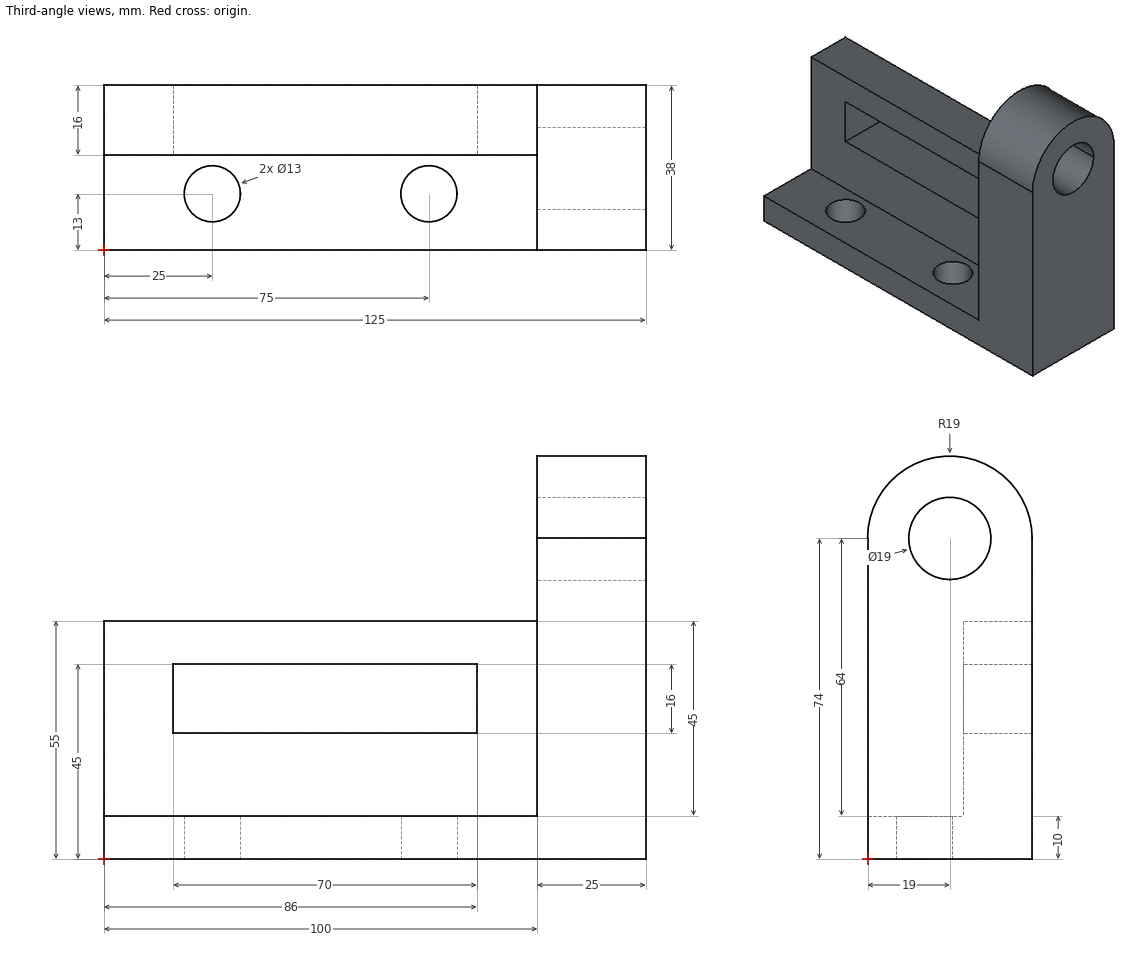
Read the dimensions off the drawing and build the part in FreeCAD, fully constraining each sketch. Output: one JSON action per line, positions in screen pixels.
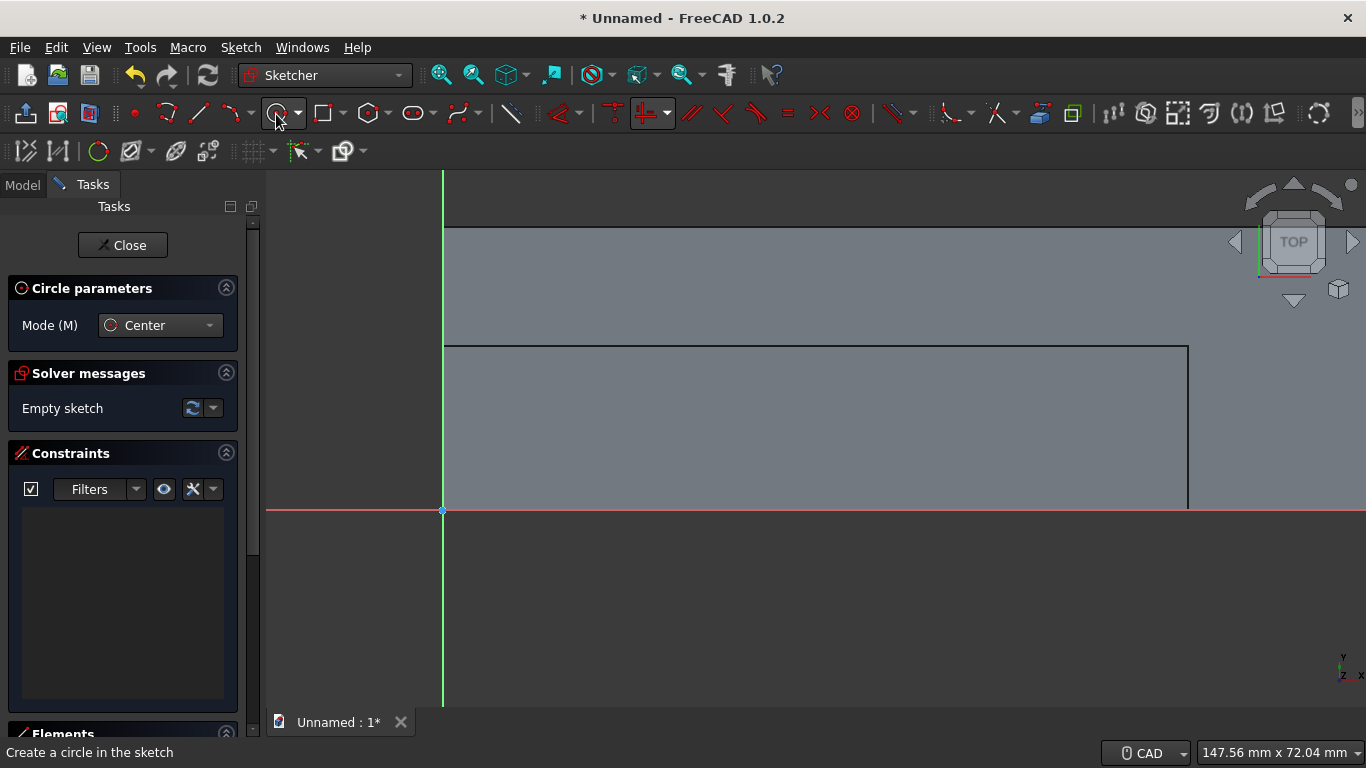
{"action": "left_click", "coordinate": [629, 413]}
{"action": "left_click", "coordinate": [663, 379]}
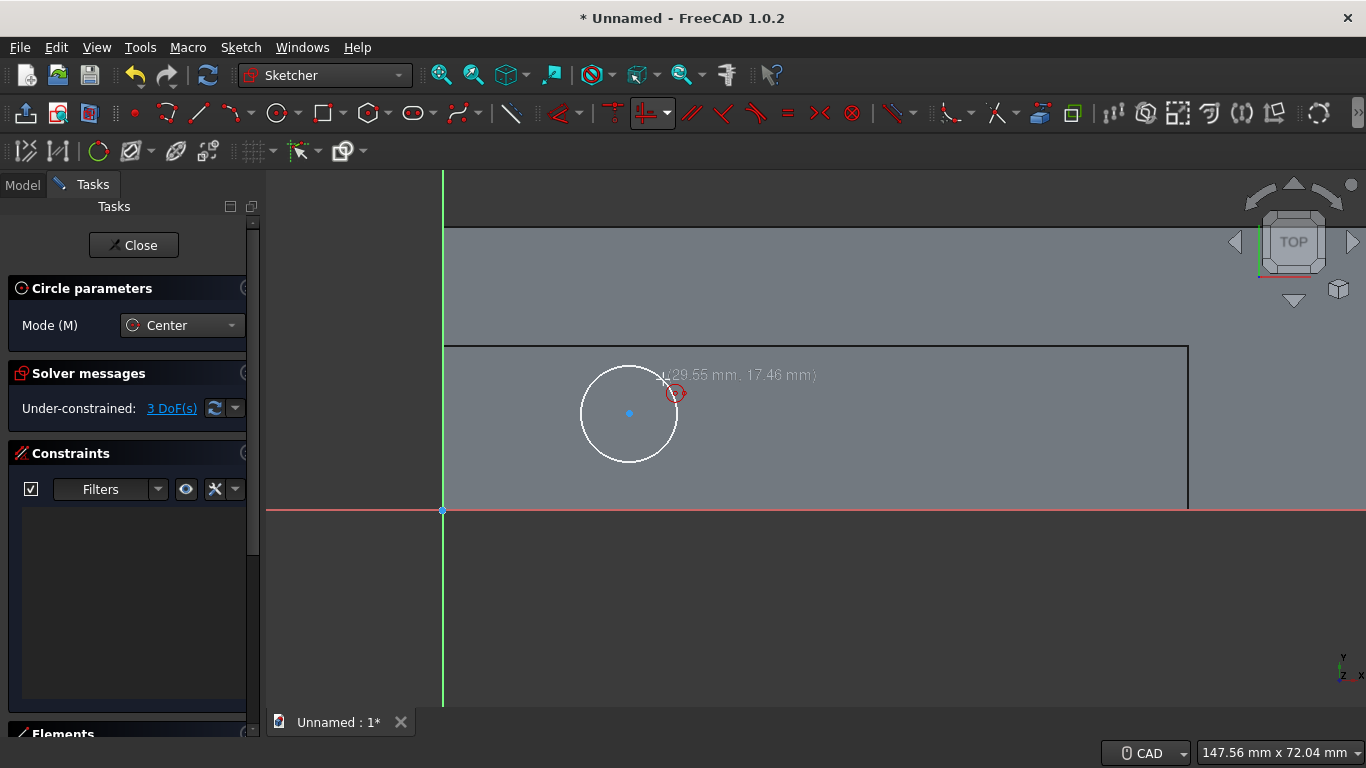
{"action": "left_click", "coordinate": [1002, 413]}
{"action": "left_click", "coordinate": [1036, 379]}
{"action": "key", "text": "Escape"}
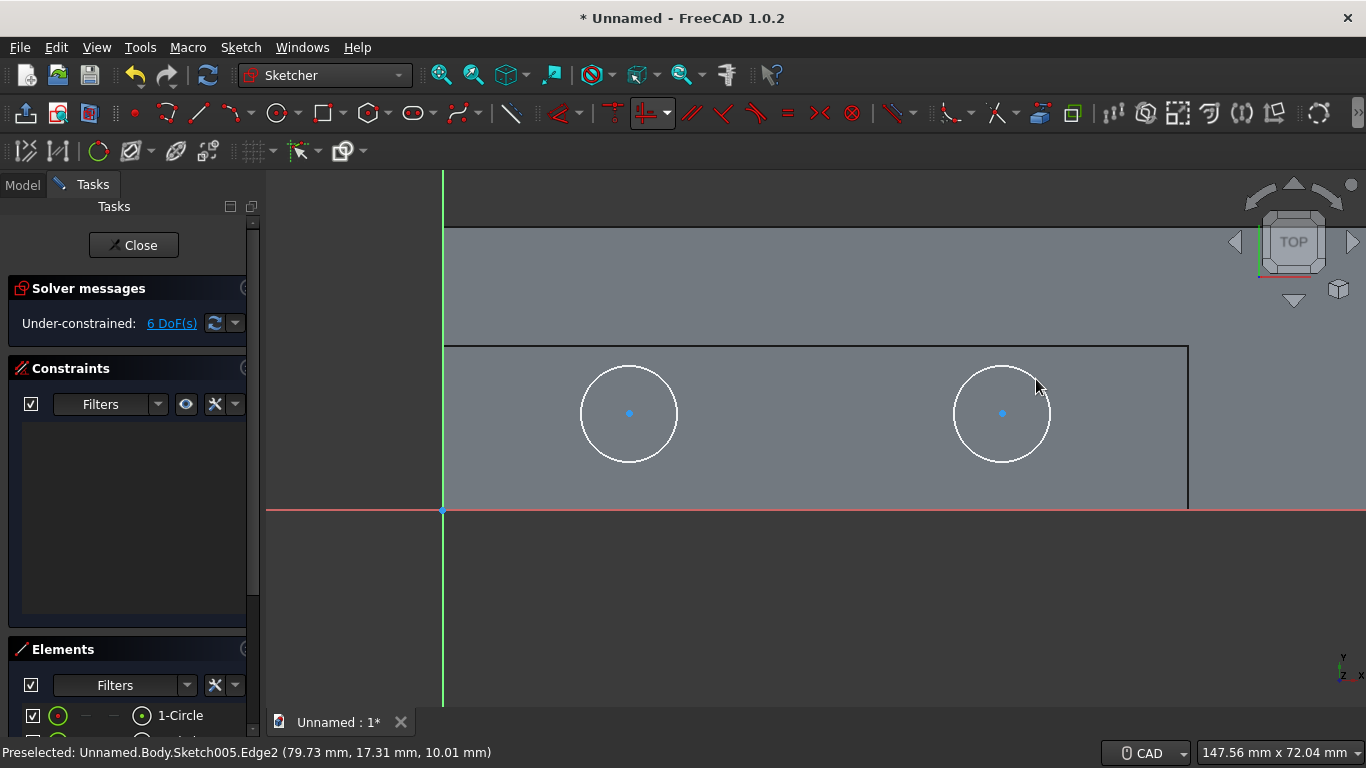
{"action": "left_click", "coordinate": [663, 380]}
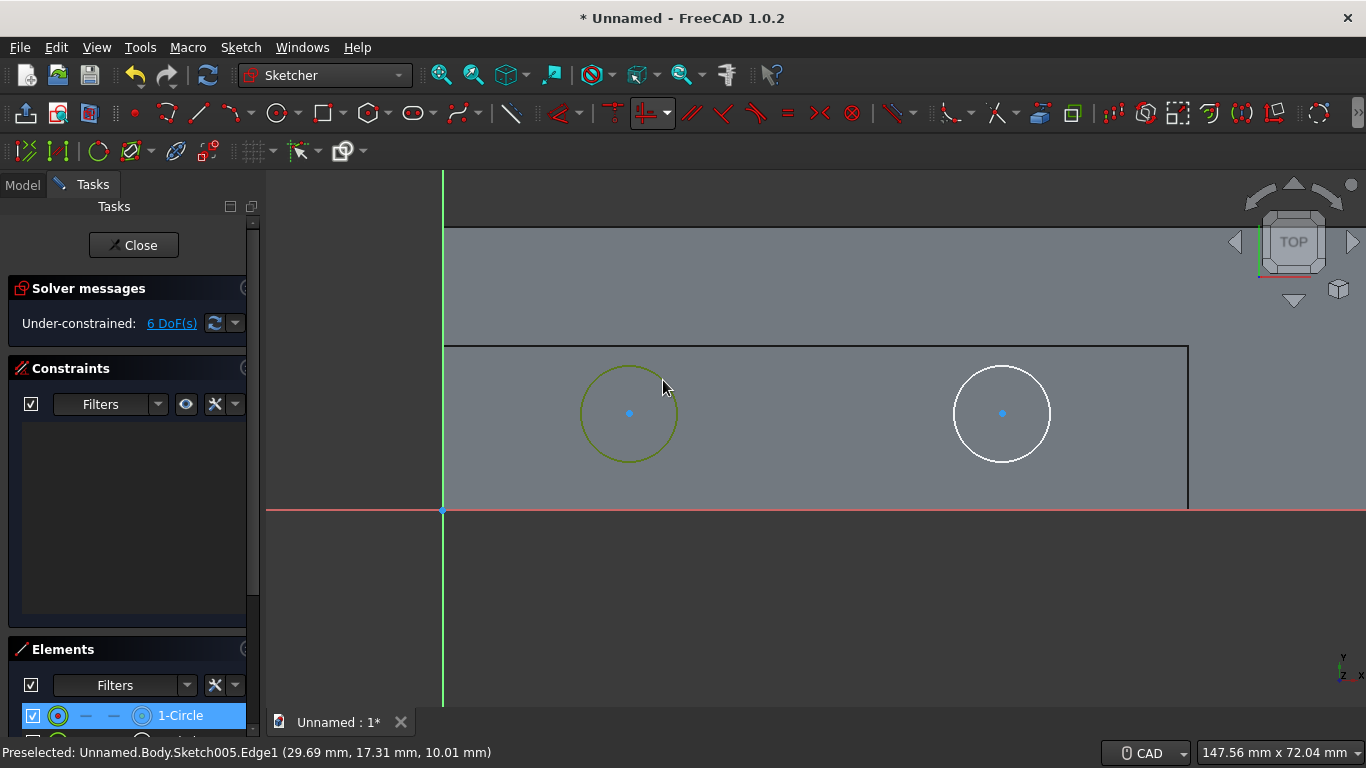
{"action": "left_click", "coordinate": [1036, 380]}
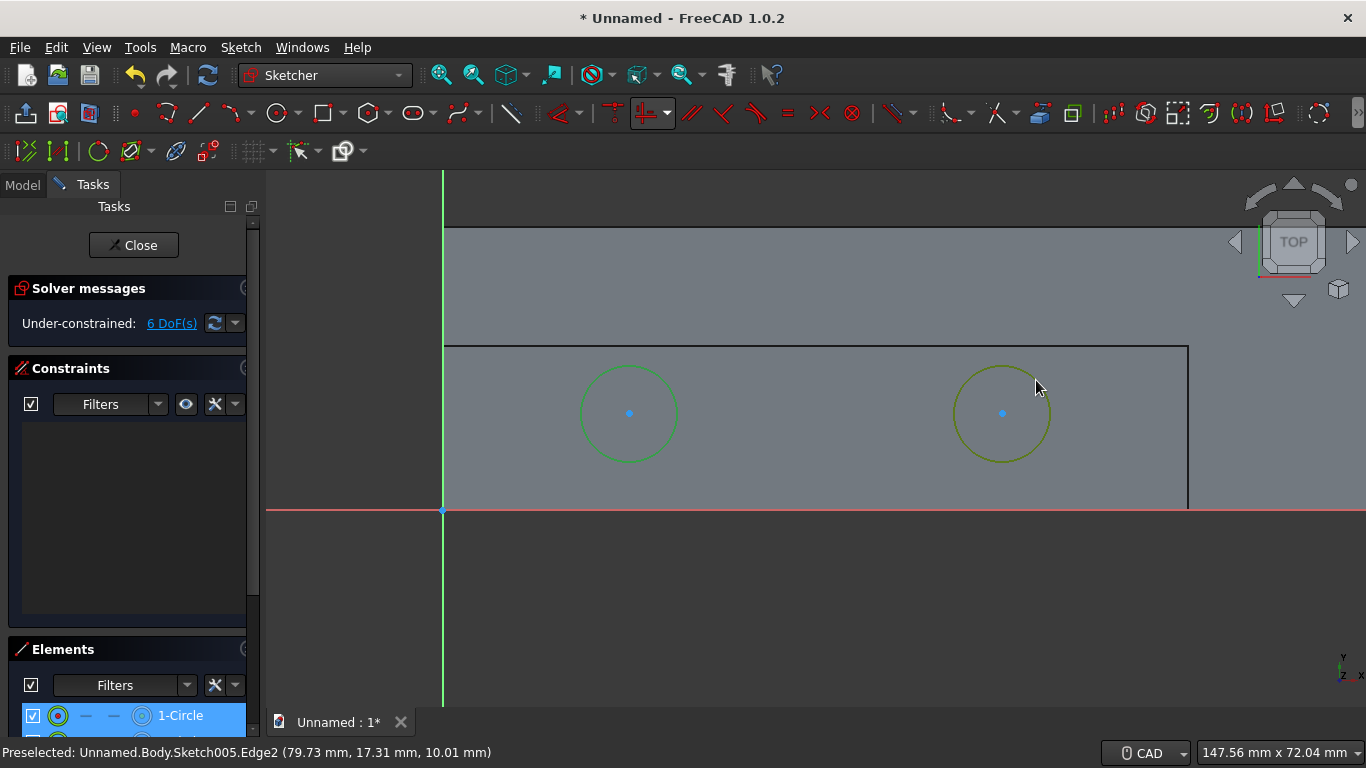
{"action": "left_click", "coordinate": [788, 114]}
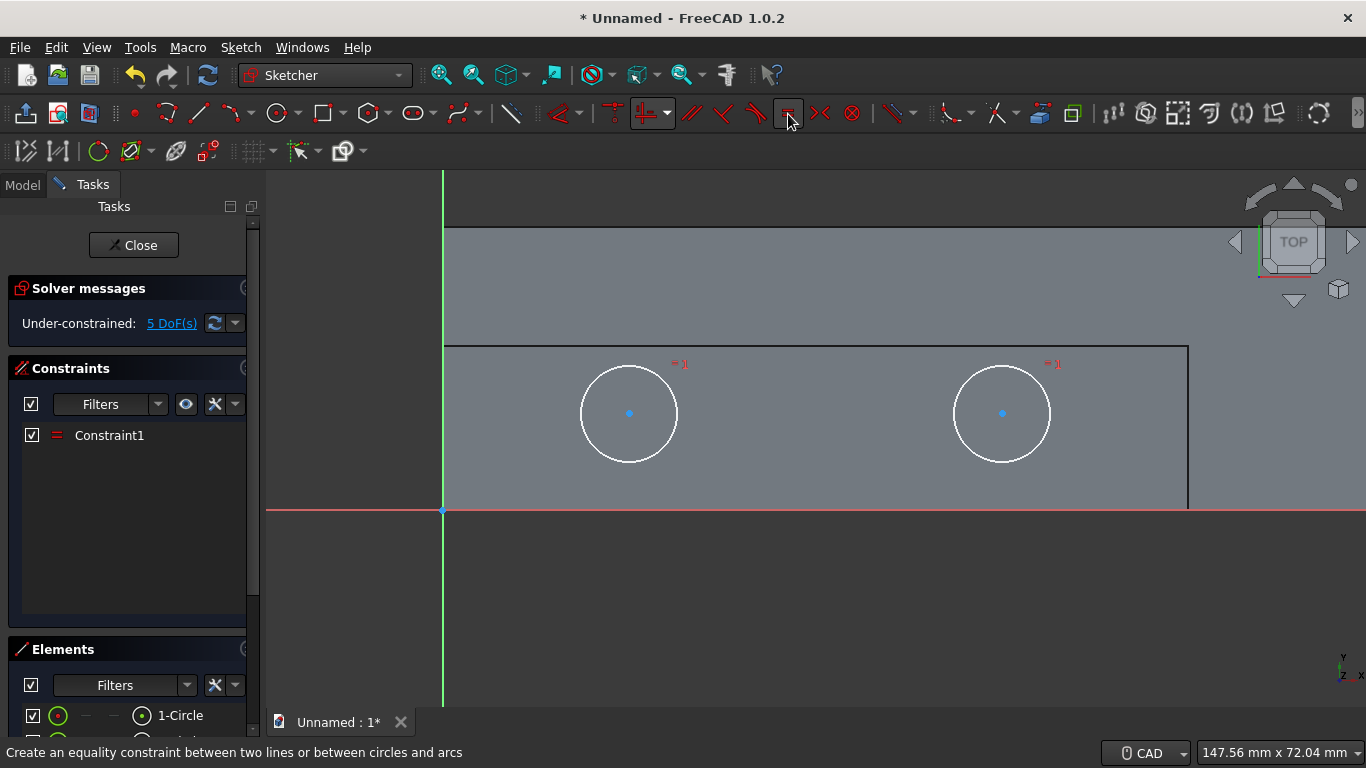
{"action": "left_click", "coordinate": [629, 414]}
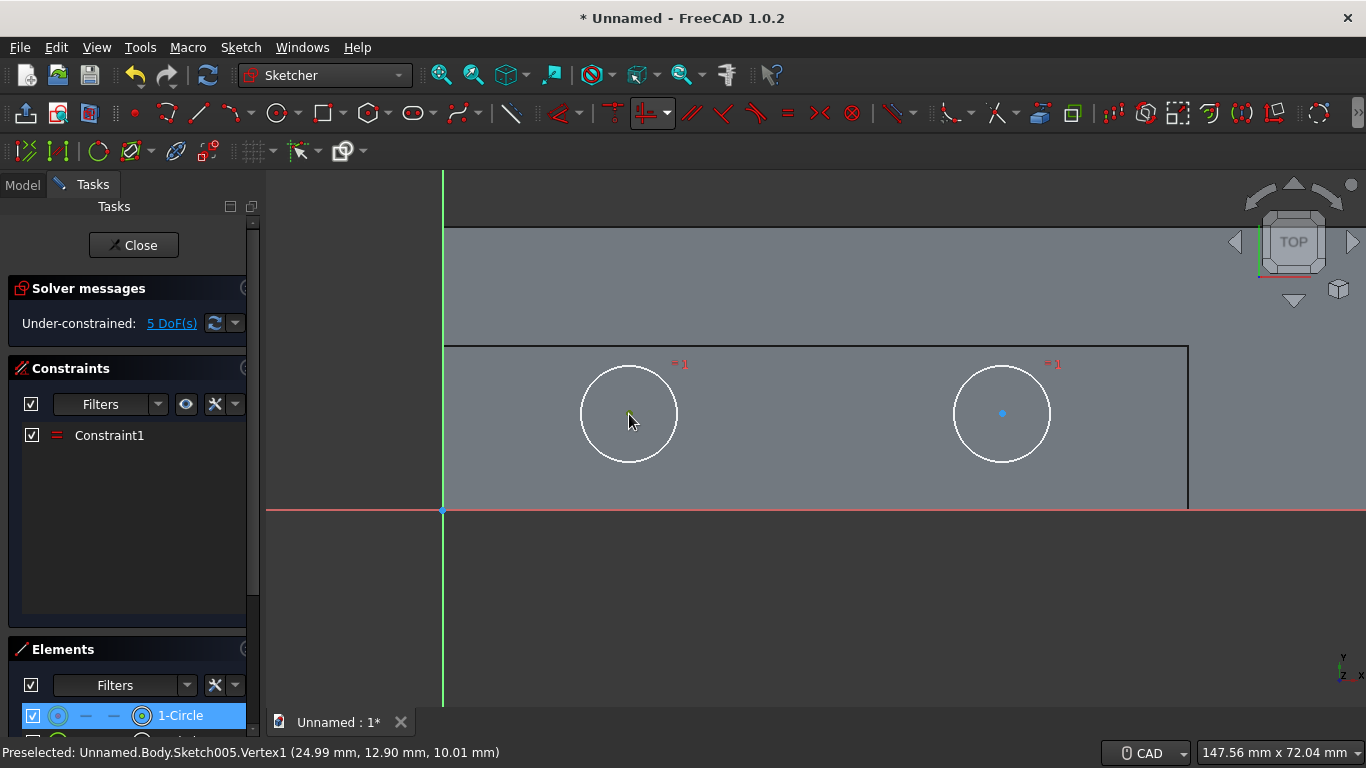
{"action": "left_click", "coordinate": [1002, 414]}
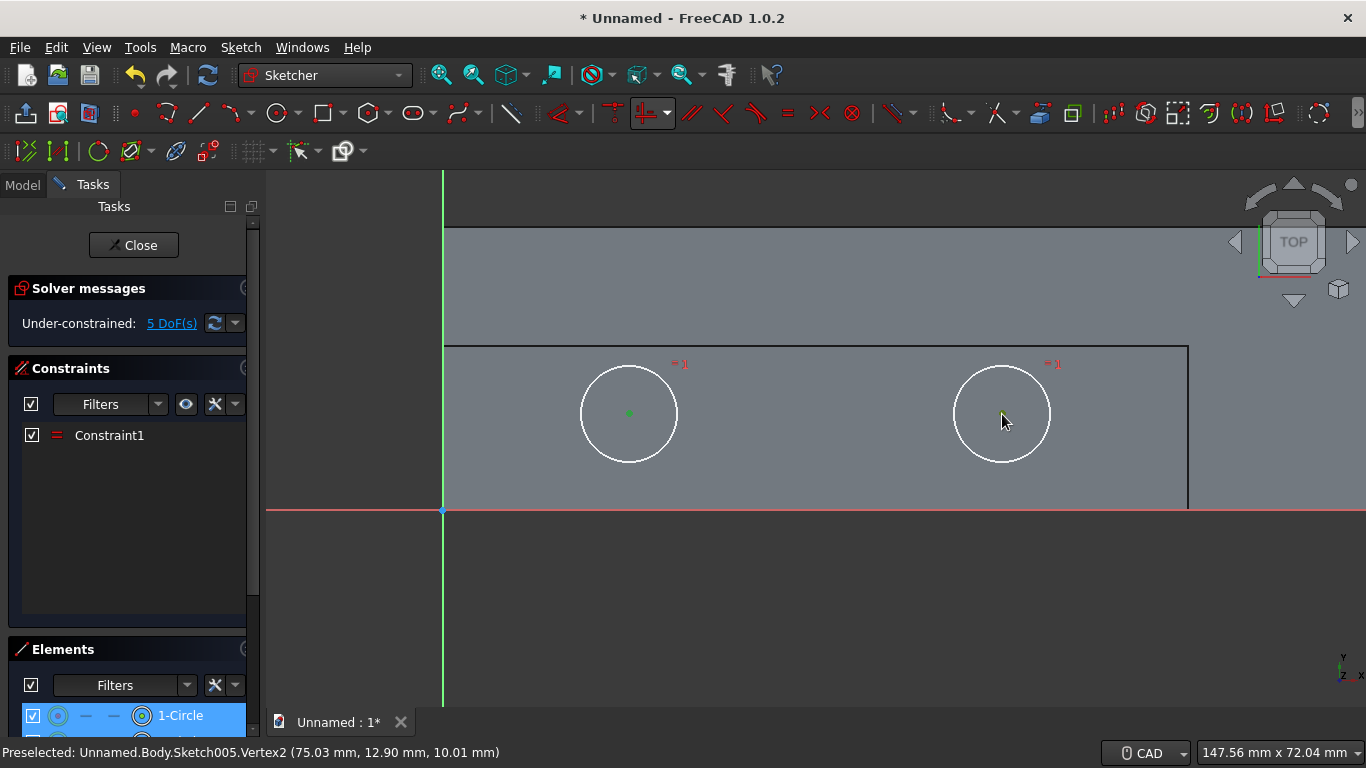
{"action": "left_click", "coordinate": [670, 114]}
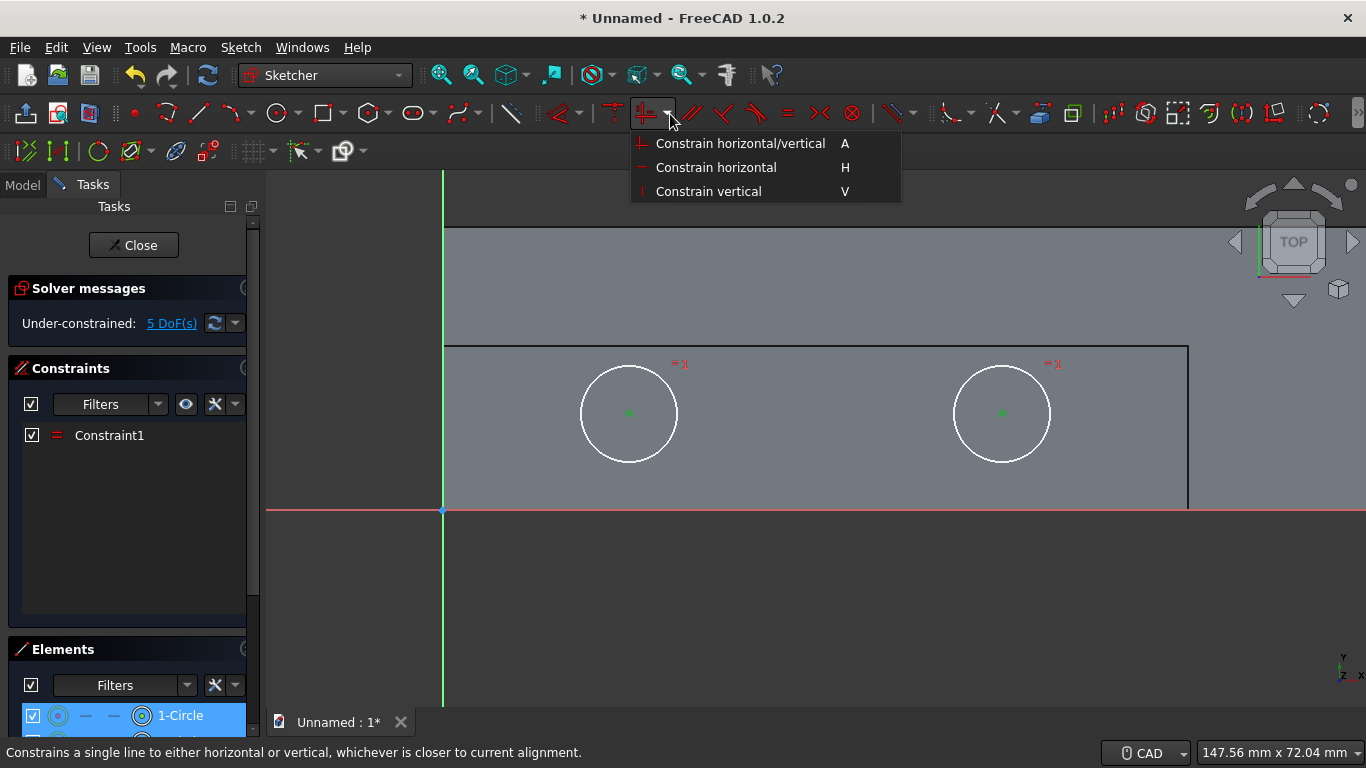
{"action": "left_click", "coordinate": [766, 167]}